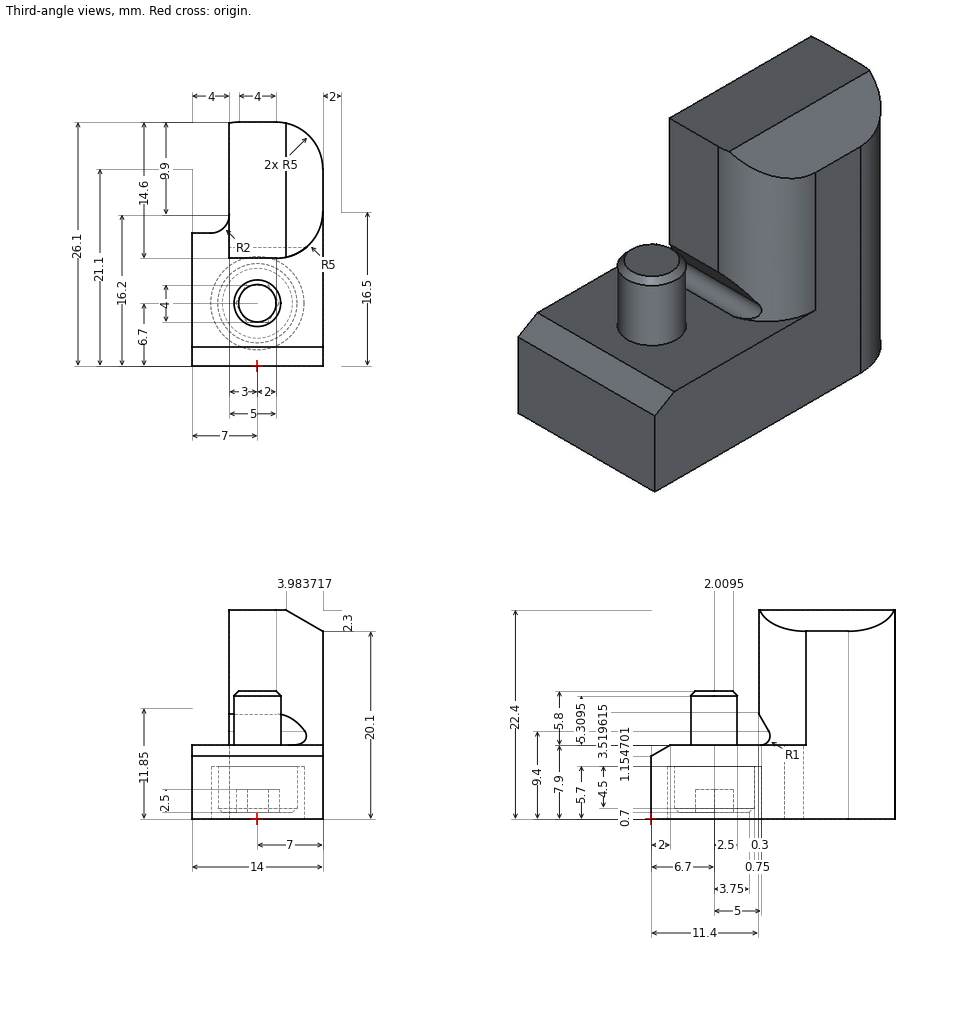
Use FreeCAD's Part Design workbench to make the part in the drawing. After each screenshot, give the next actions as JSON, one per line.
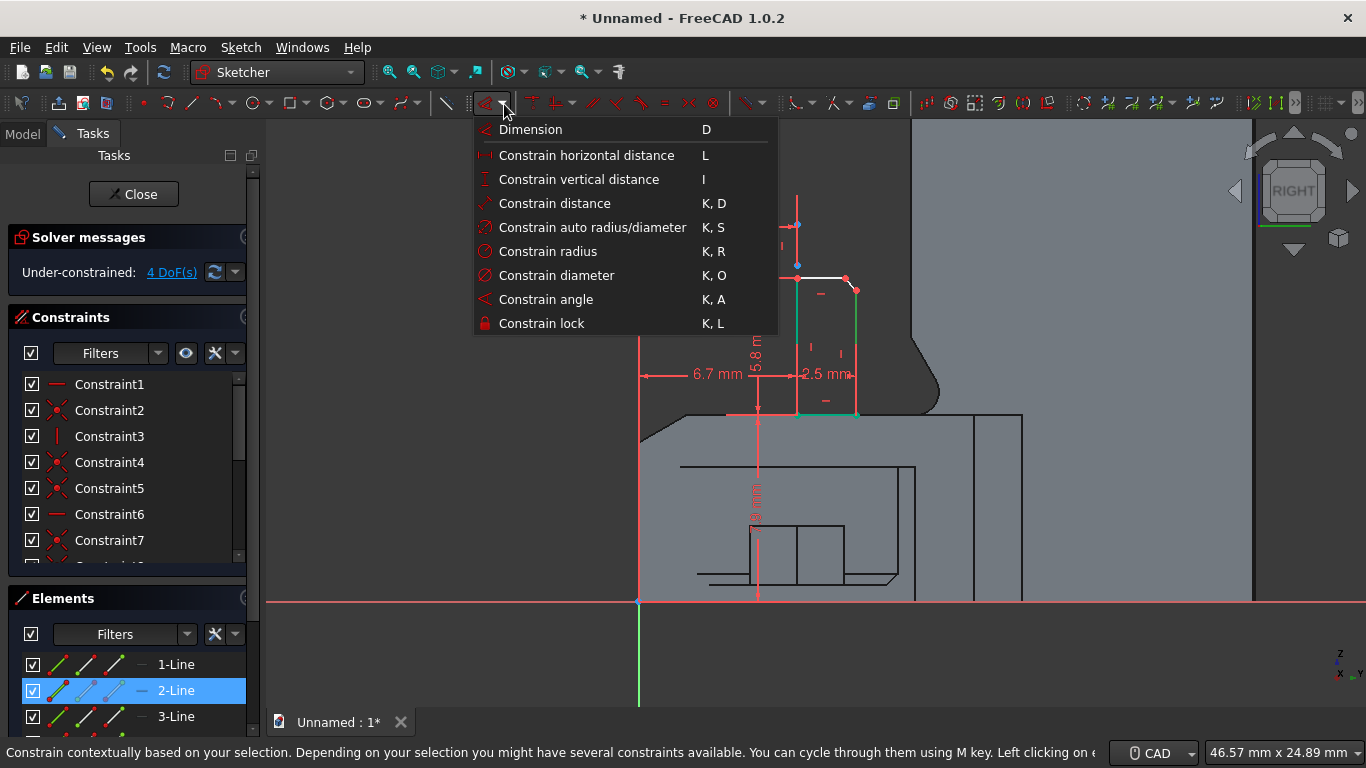
{"action": "left_click", "coordinate": [626, 179]}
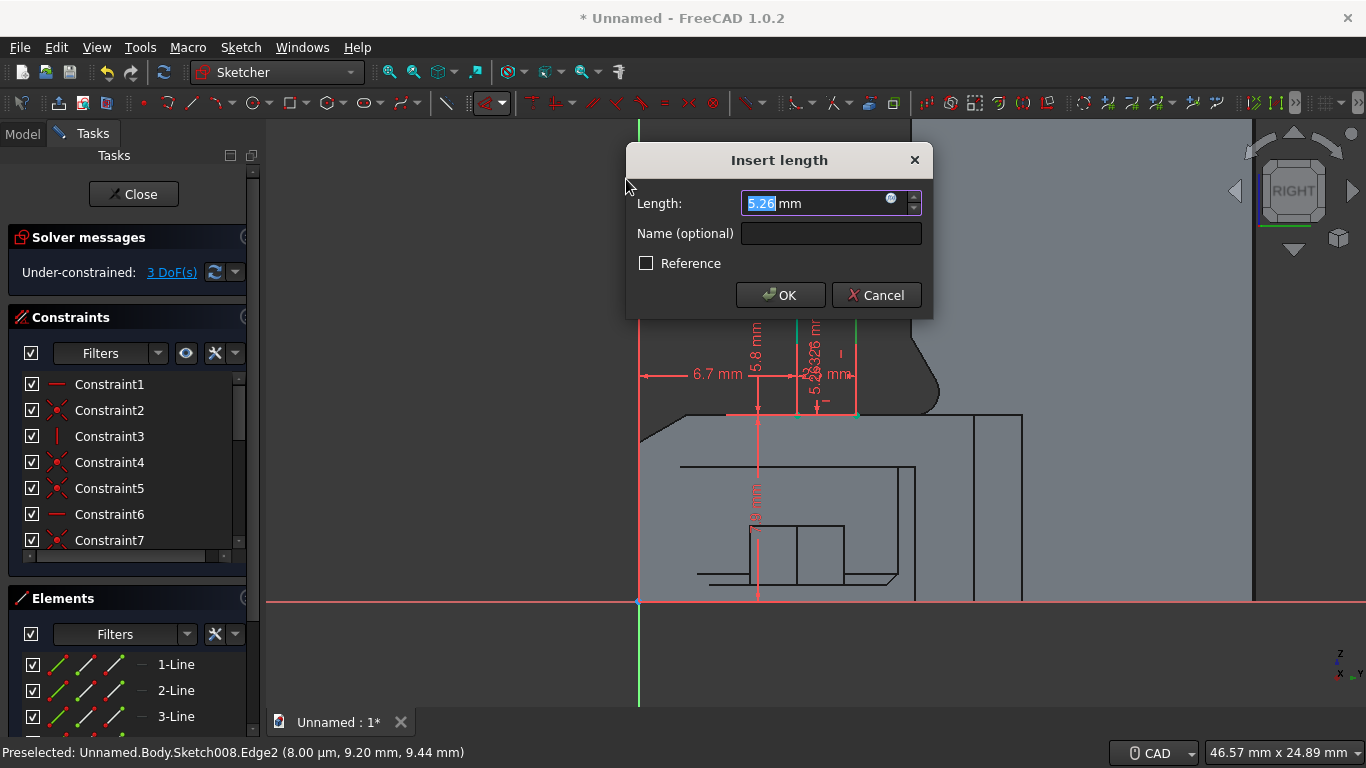
{"action": "type", "text": "5.3095"}
{"action": "key", "text": "Return"}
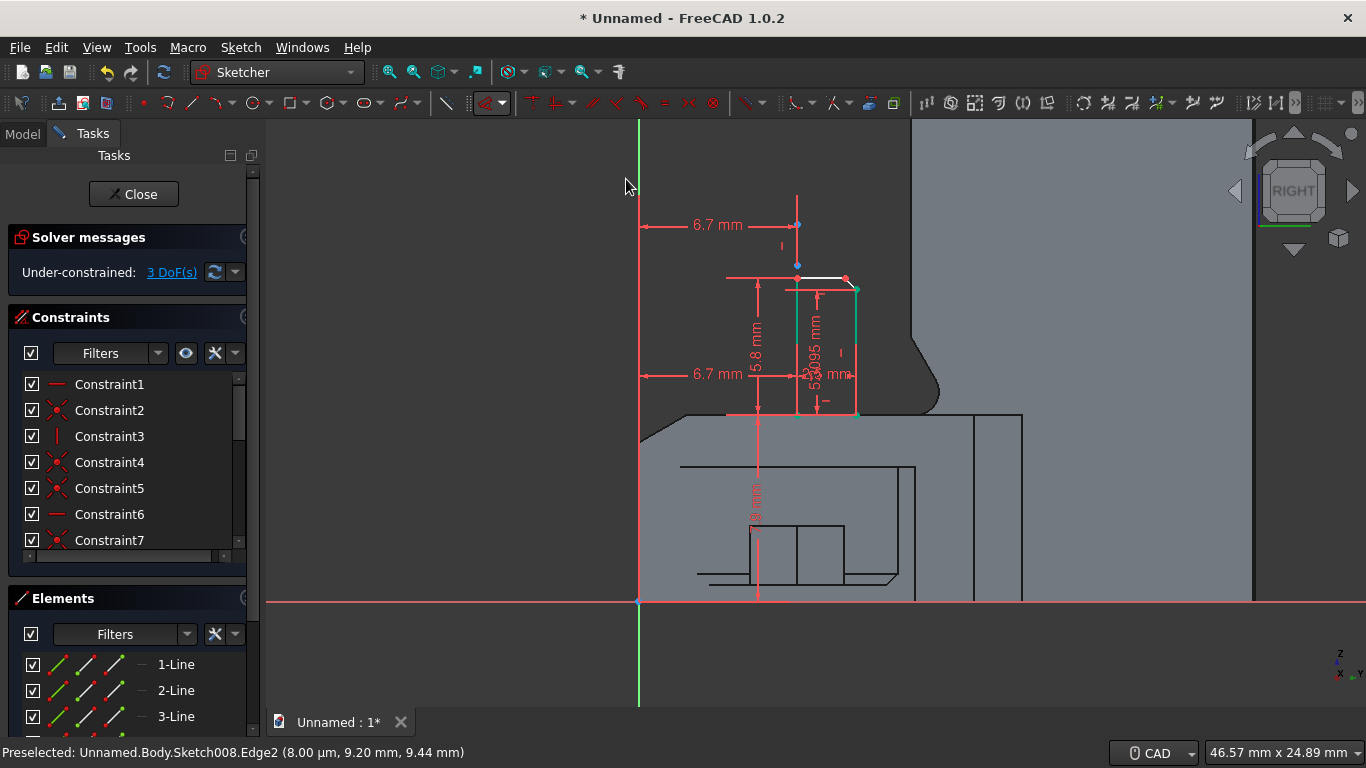
{"action": "left_click", "coordinate": [831, 278]}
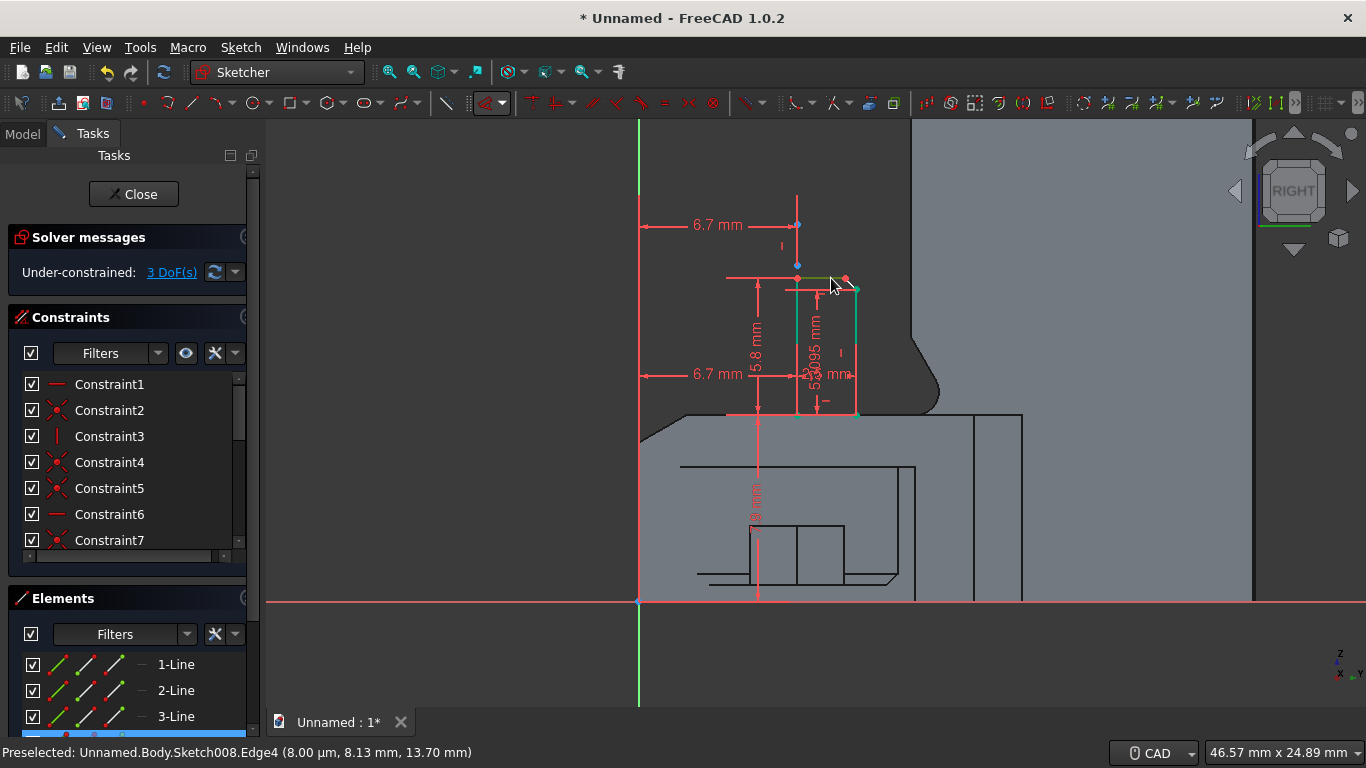
{"action": "left_click", "coordinate": [504, 104]}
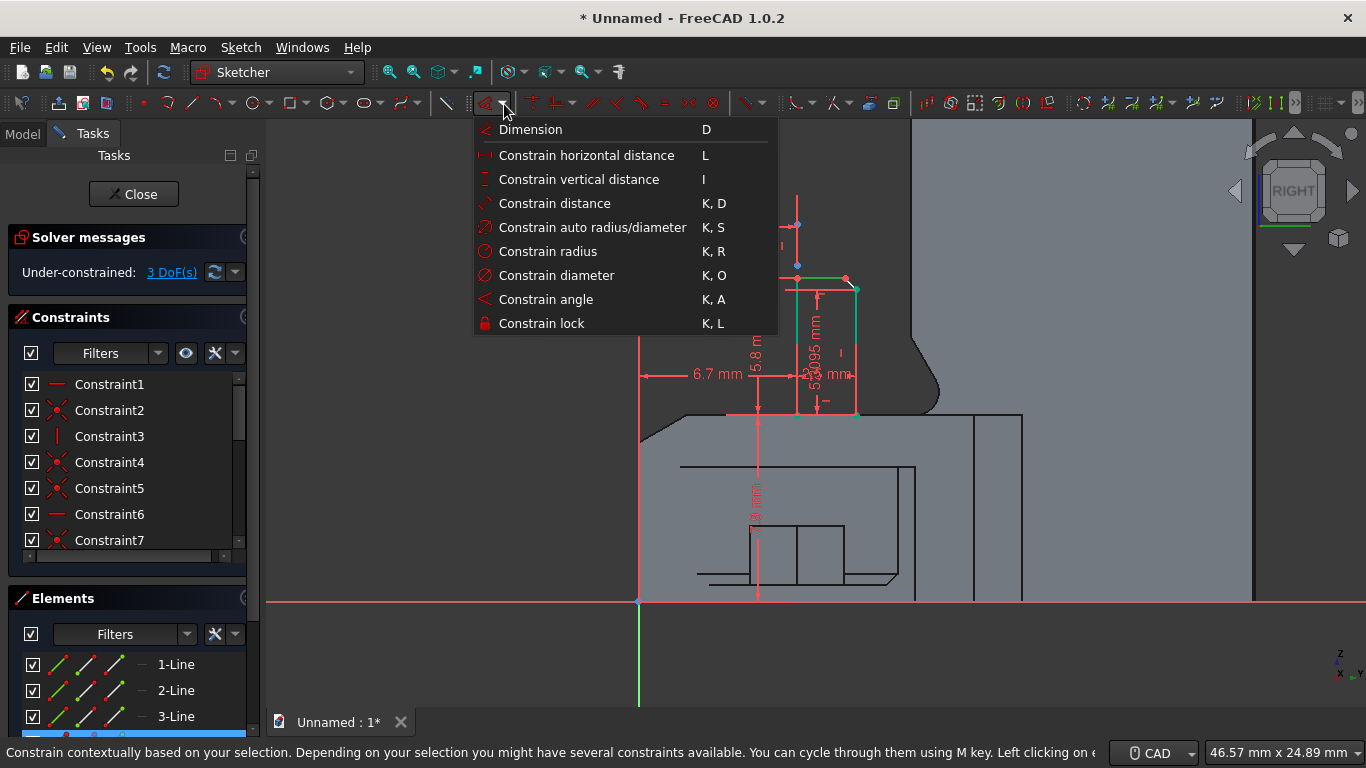
{"action": "left_click", "coordinate": [626, 155]}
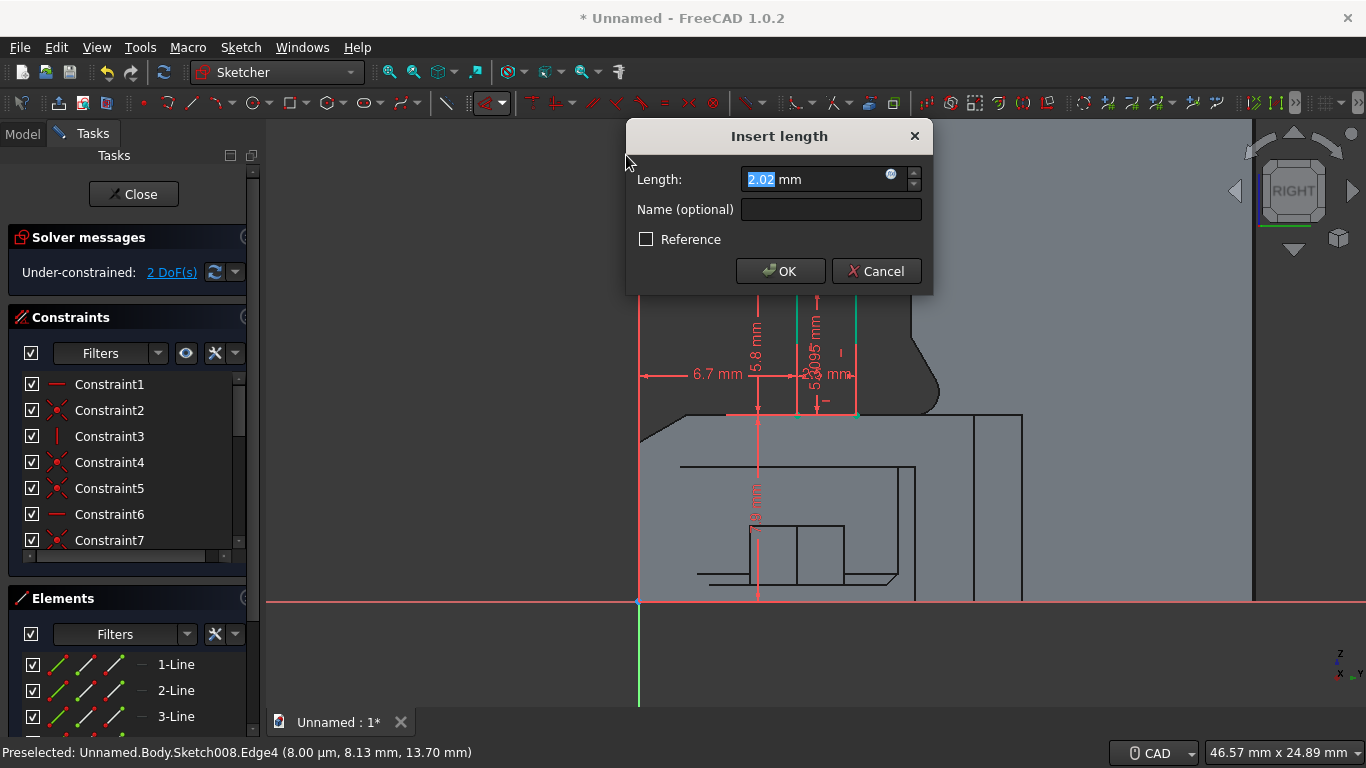
{"action": "type", "text": "2.0095"}
{"action": "key", "text": "Return"}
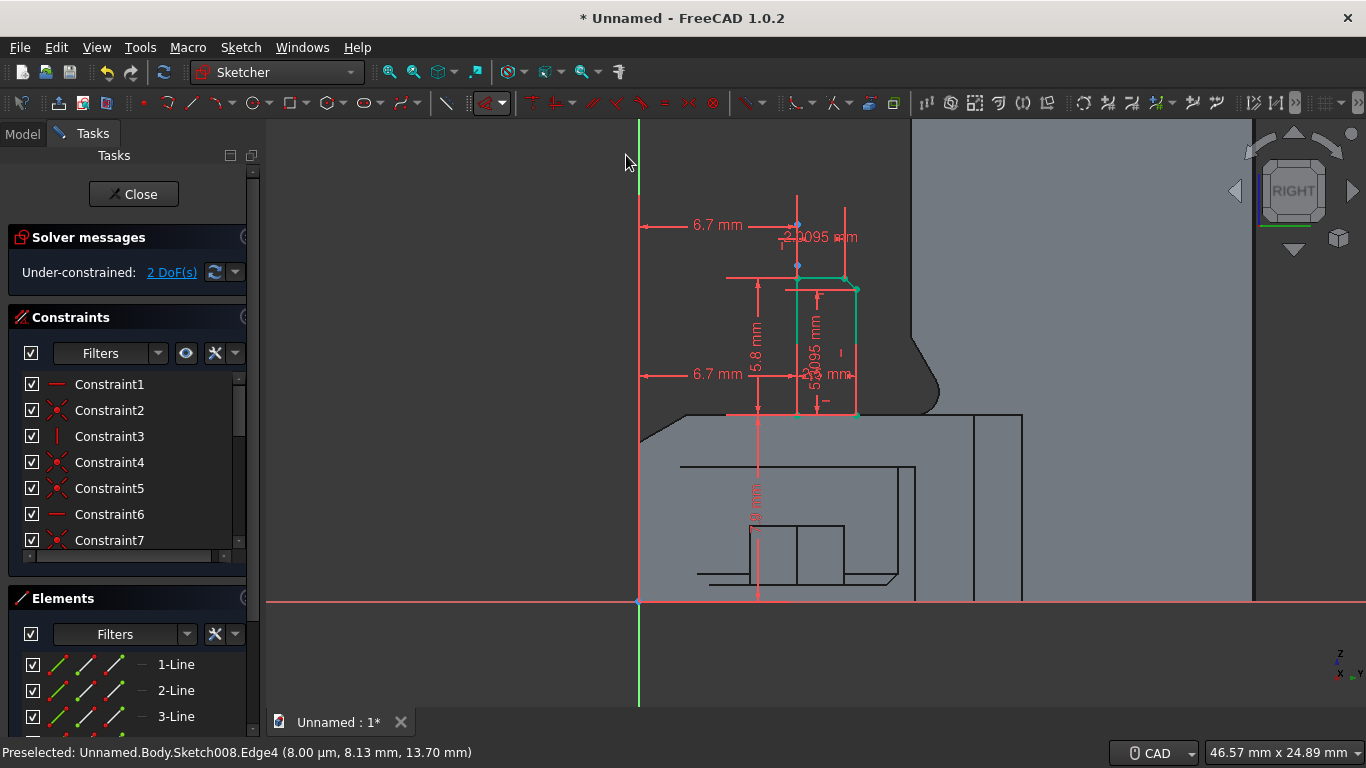
{"action": "left_click", "coordinate": [134, 194]}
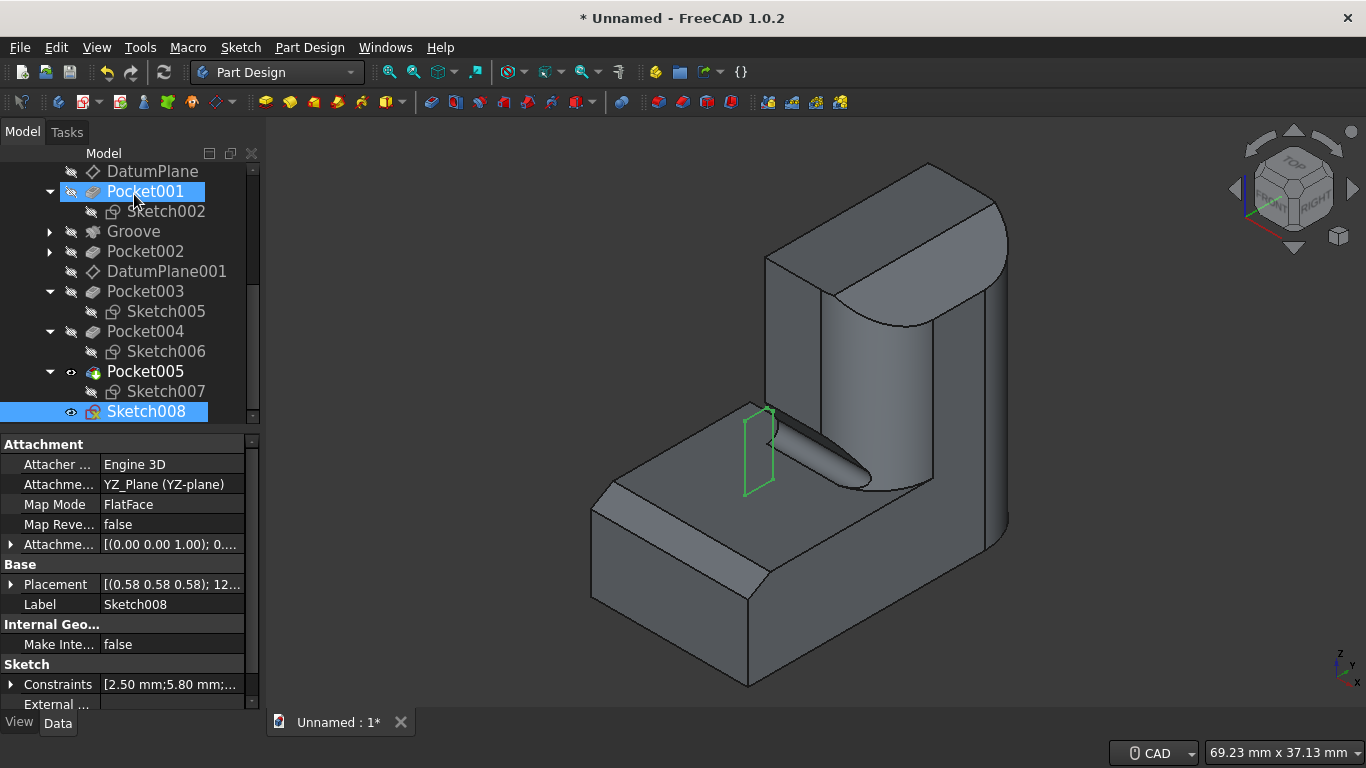
{"action": "left_click", "coordinate": [290, 102]}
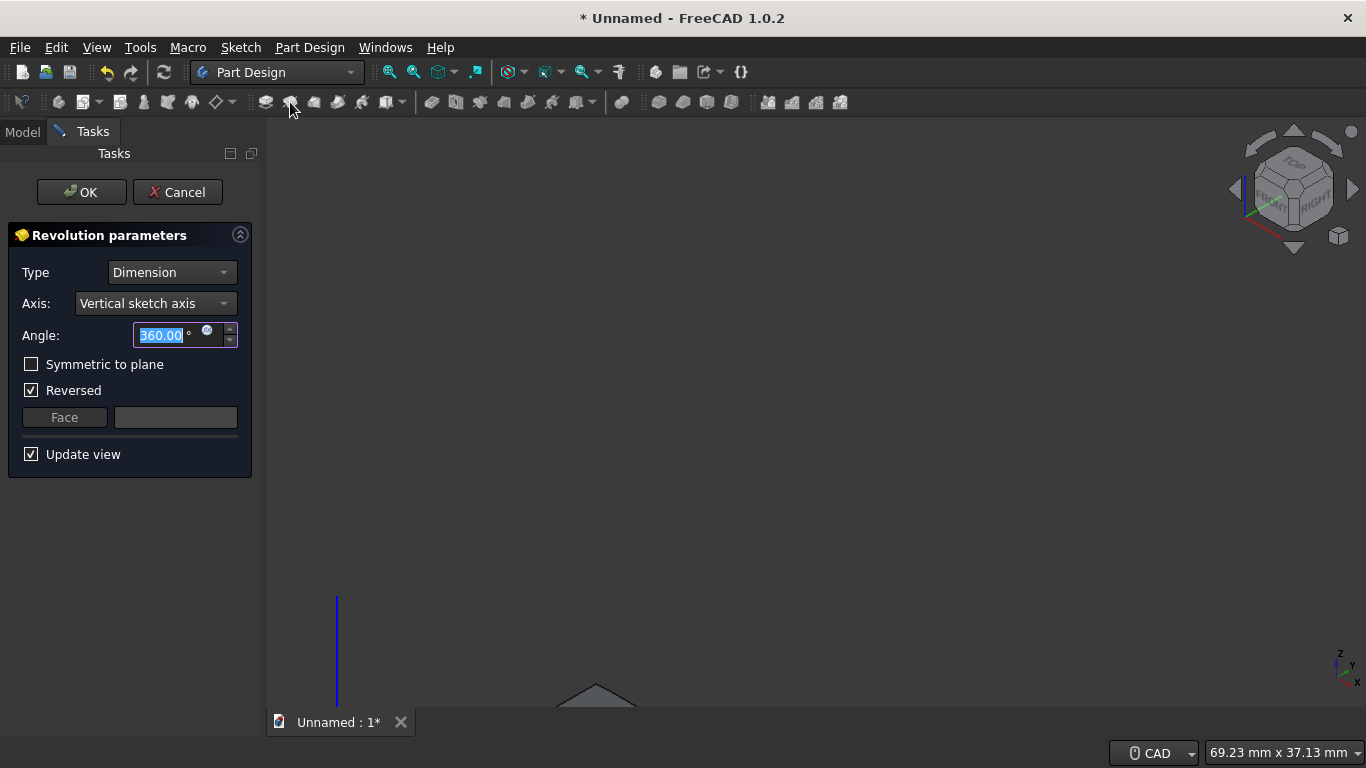
{"action": "left_click", "coordinate": [156, 304]}